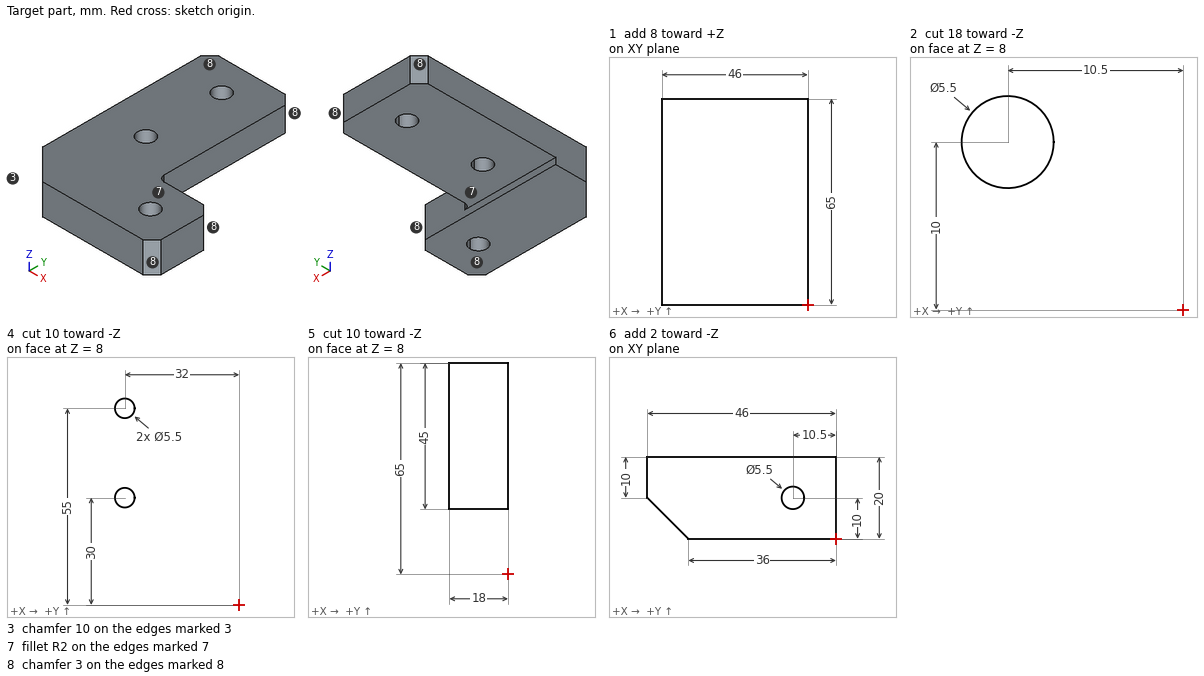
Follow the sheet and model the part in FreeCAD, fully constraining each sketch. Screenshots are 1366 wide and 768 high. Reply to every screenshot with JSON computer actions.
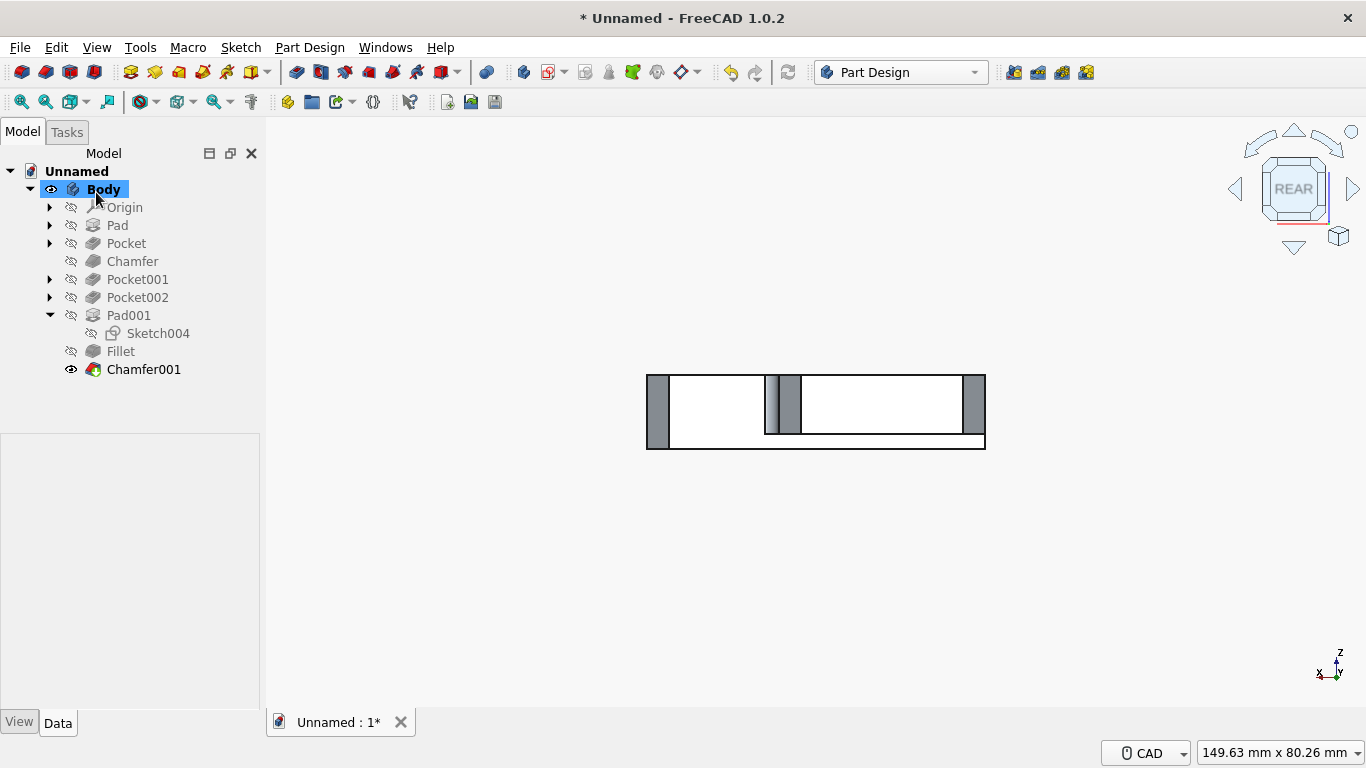
{"action": "key", "text": "0"}